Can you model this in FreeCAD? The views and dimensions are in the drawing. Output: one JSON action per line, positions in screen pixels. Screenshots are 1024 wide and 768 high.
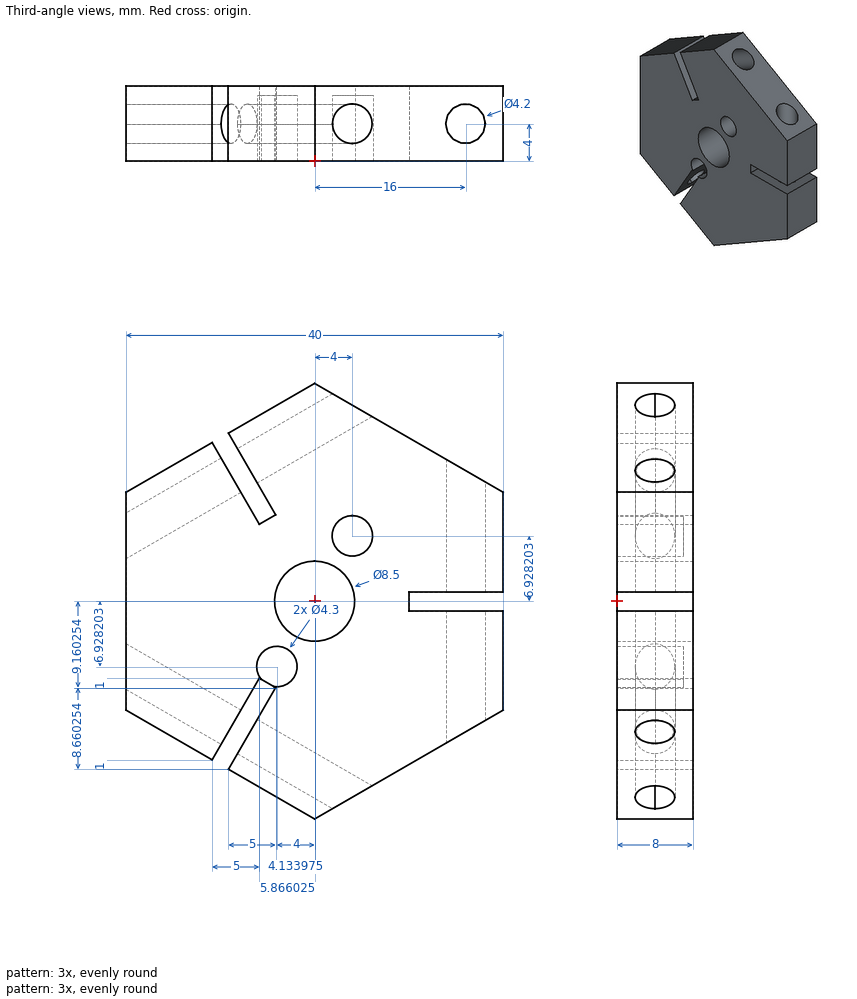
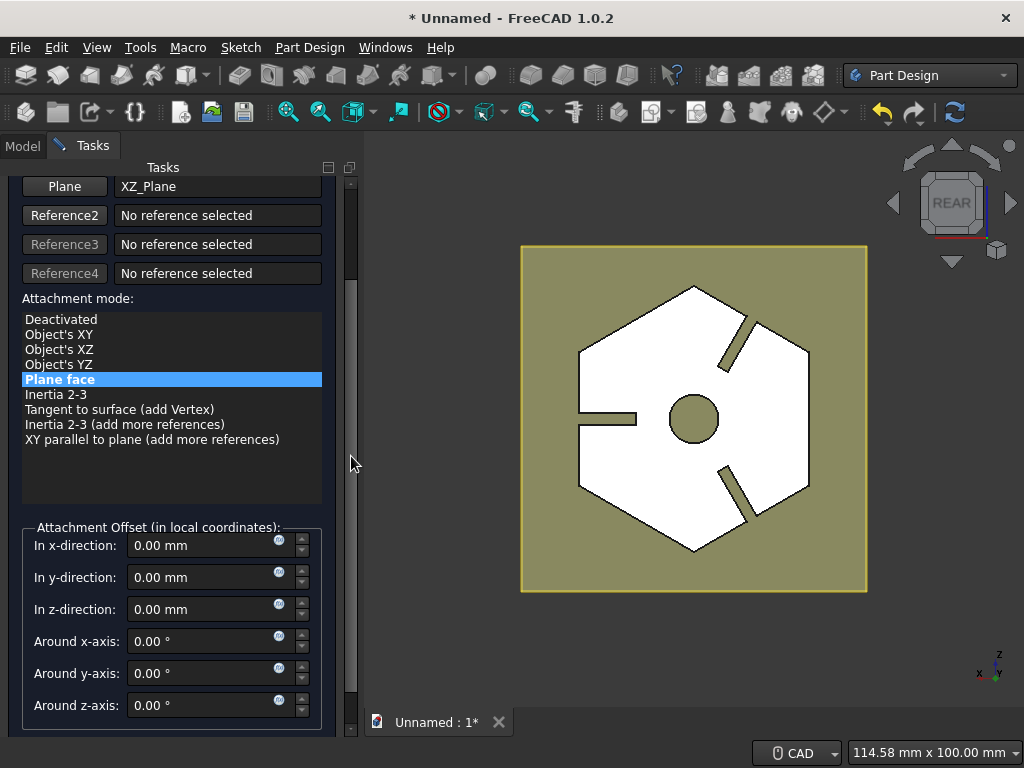
{"action": "triple_click", "coordinate": [210, 609]}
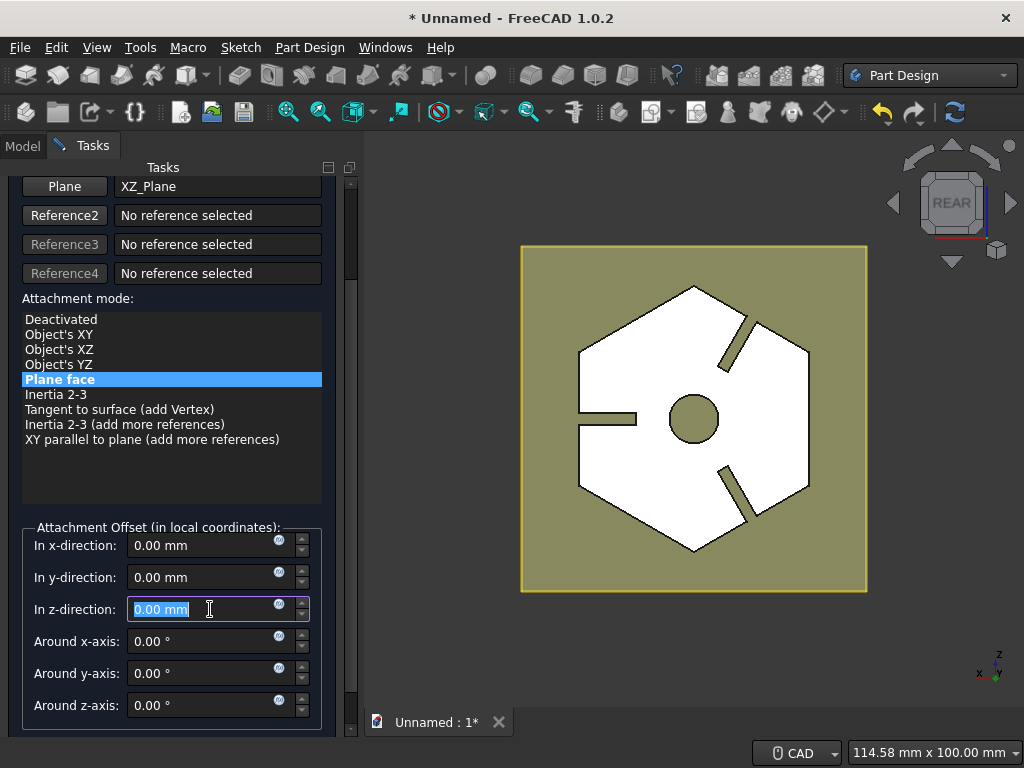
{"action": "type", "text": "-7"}
{"action": "key", "text": "Tab"}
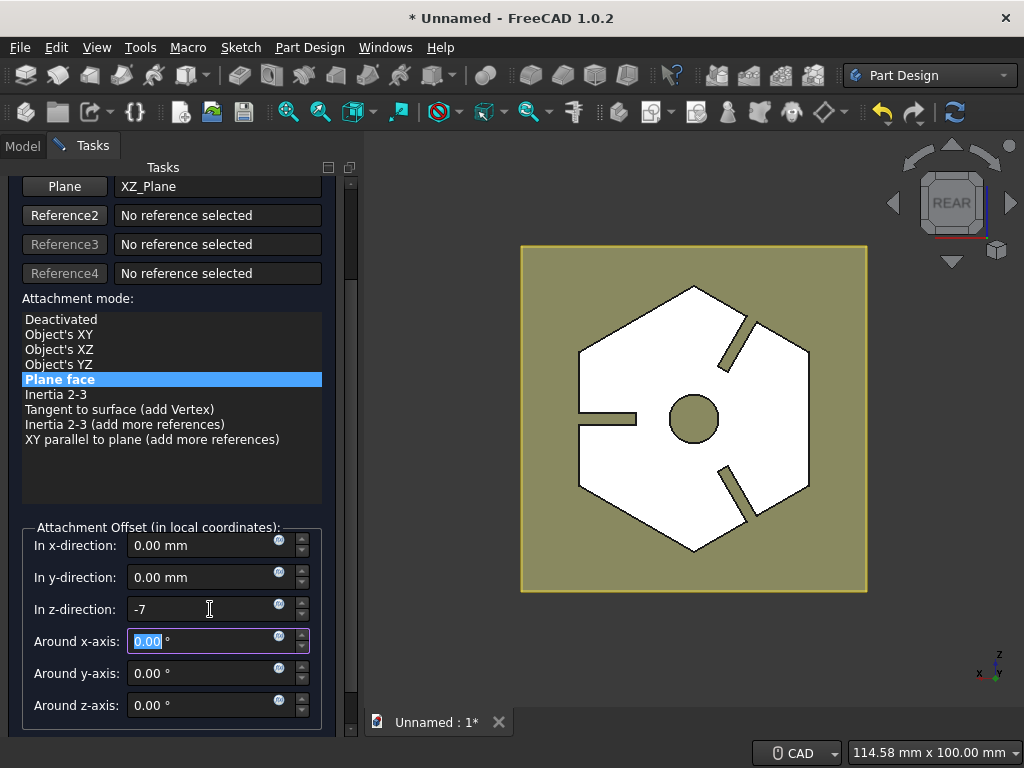
{"action": "scroll", "coordinate": [351, 456], "scroll_direction": "up", "scroll_amount": 3}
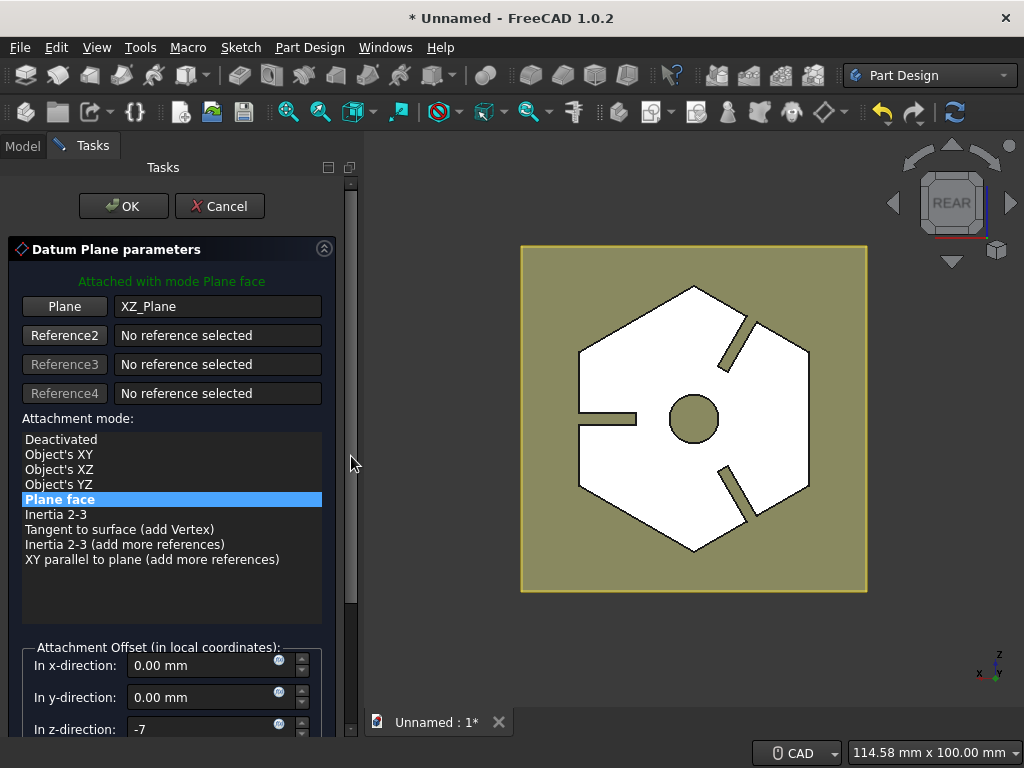
{"action": "left_click", "coordinate": [124, 206]}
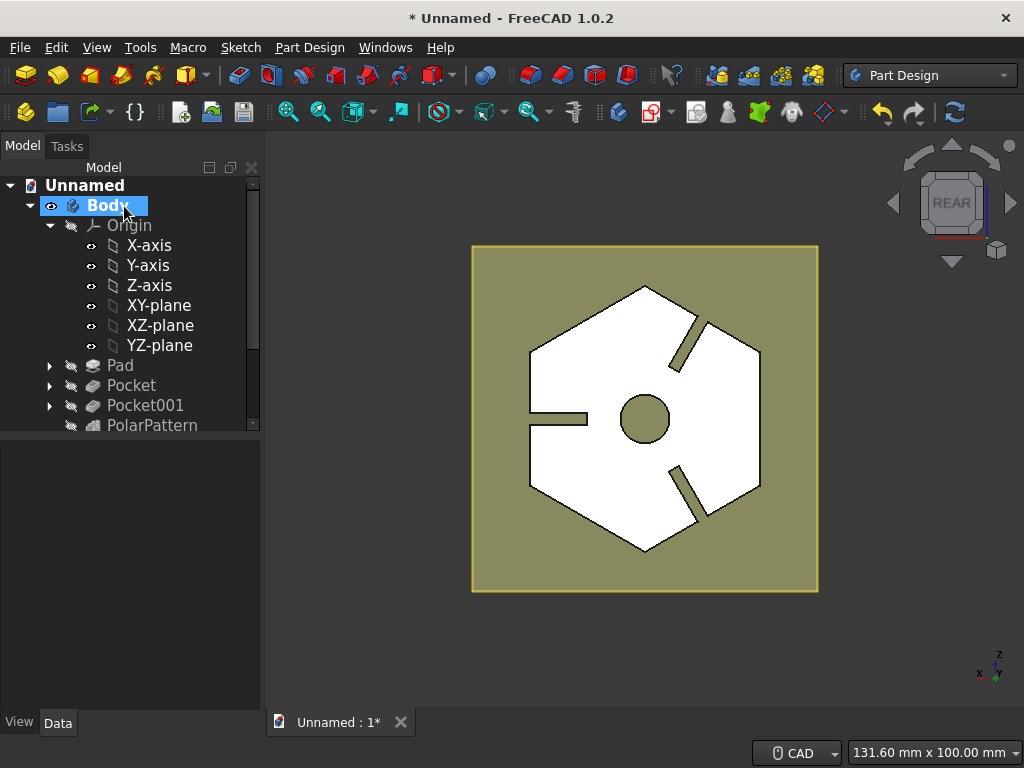
{"action": "scroll", "coordinate": [100, 301], "scroll_direction": "down", "scroll_amount": 3}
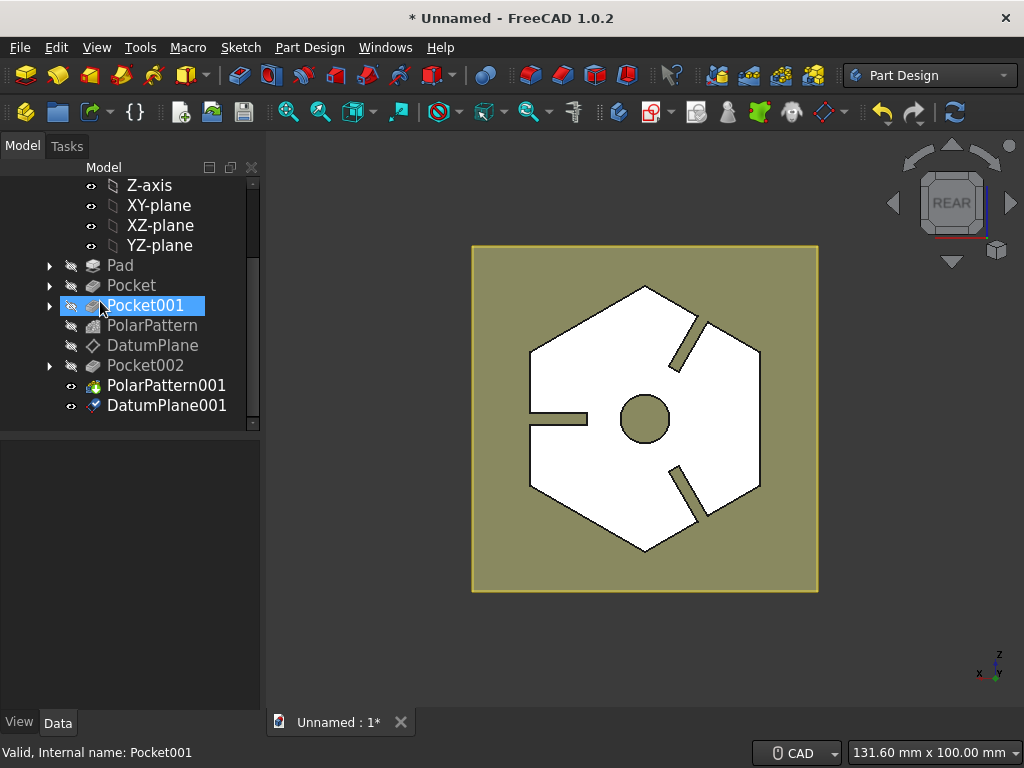
{"action": "left_click", "coordinate": [116, 406]}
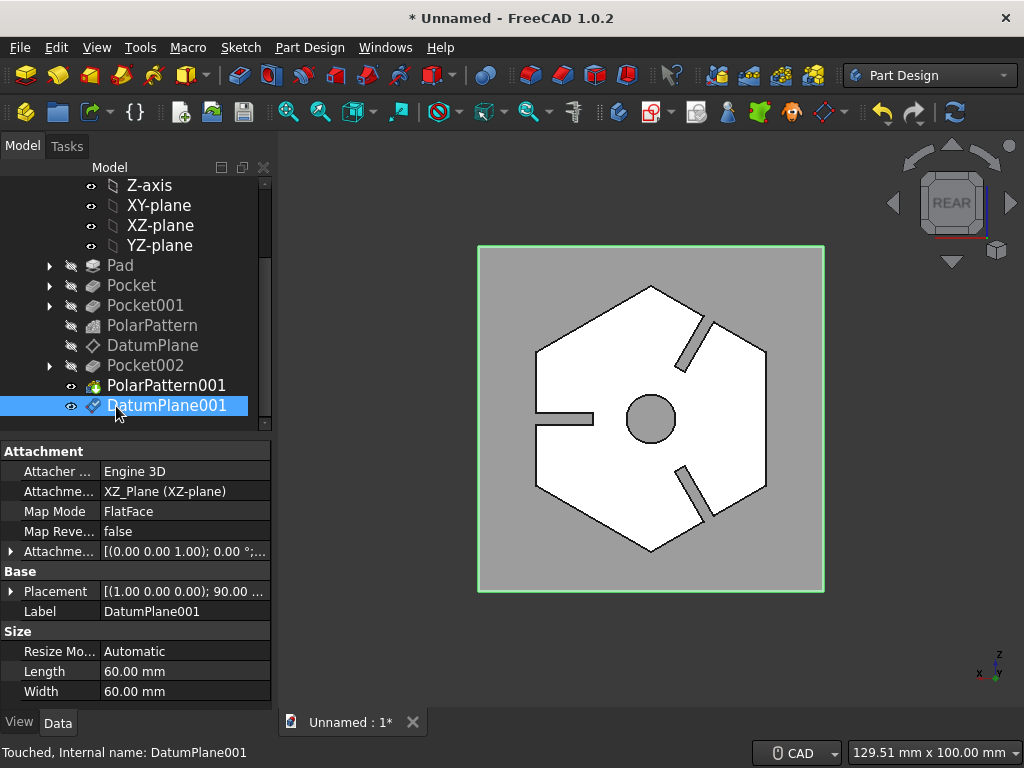
{"action": "left_click", "coordinate": [652, 112]}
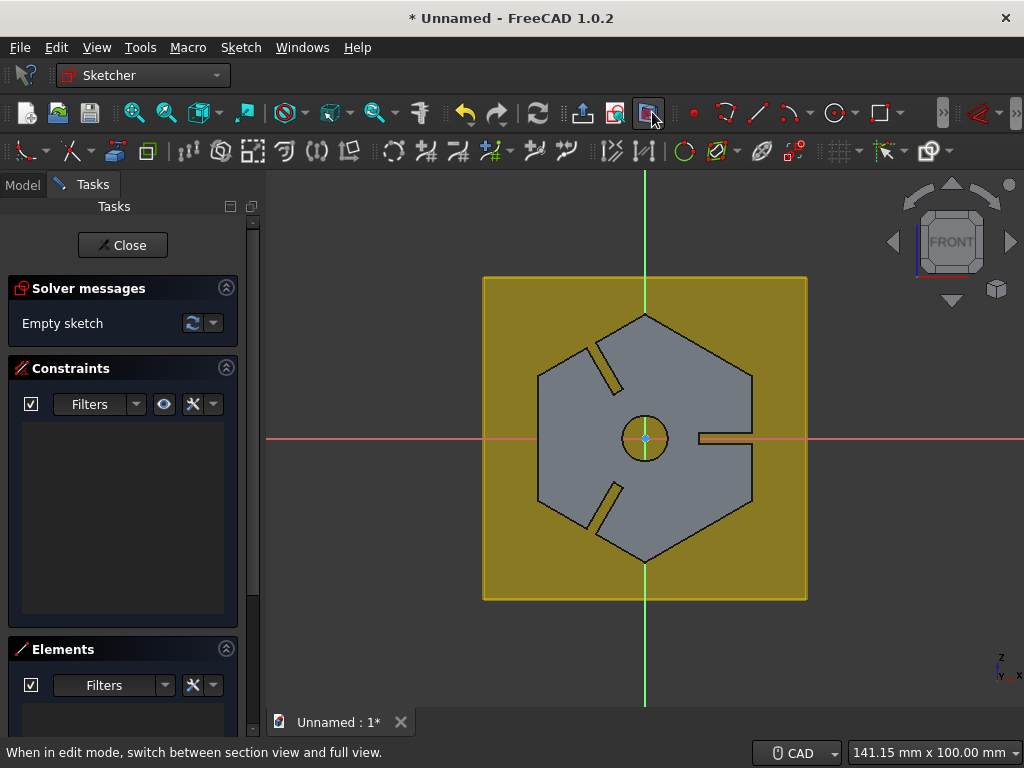
{"action": "key", "text": "q s"}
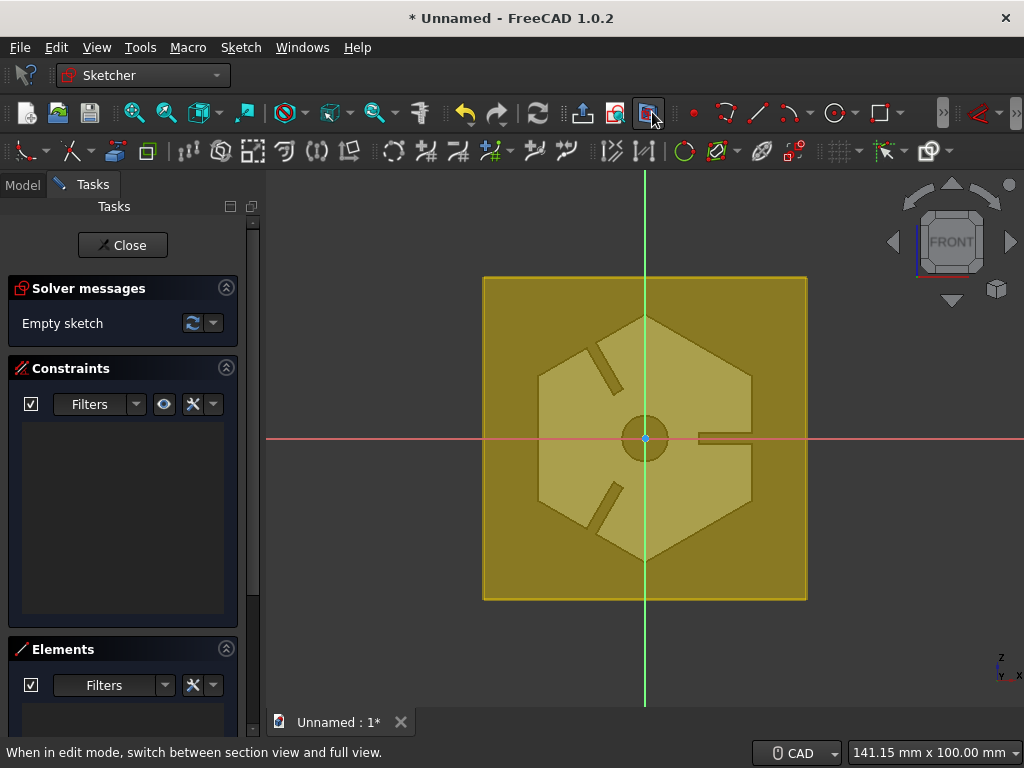
{"action": "scroll", "coordinate": [675, 439], "scroll_direction": "up", "scroll_amount": 6}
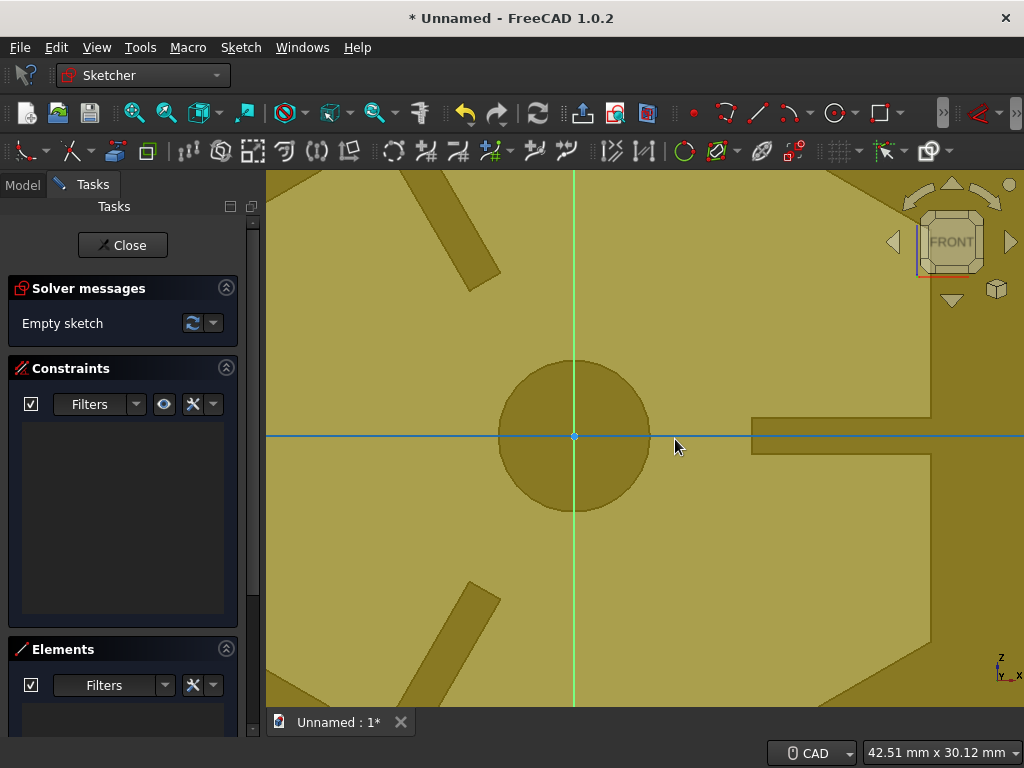
{"action": "key", "text": "g c"}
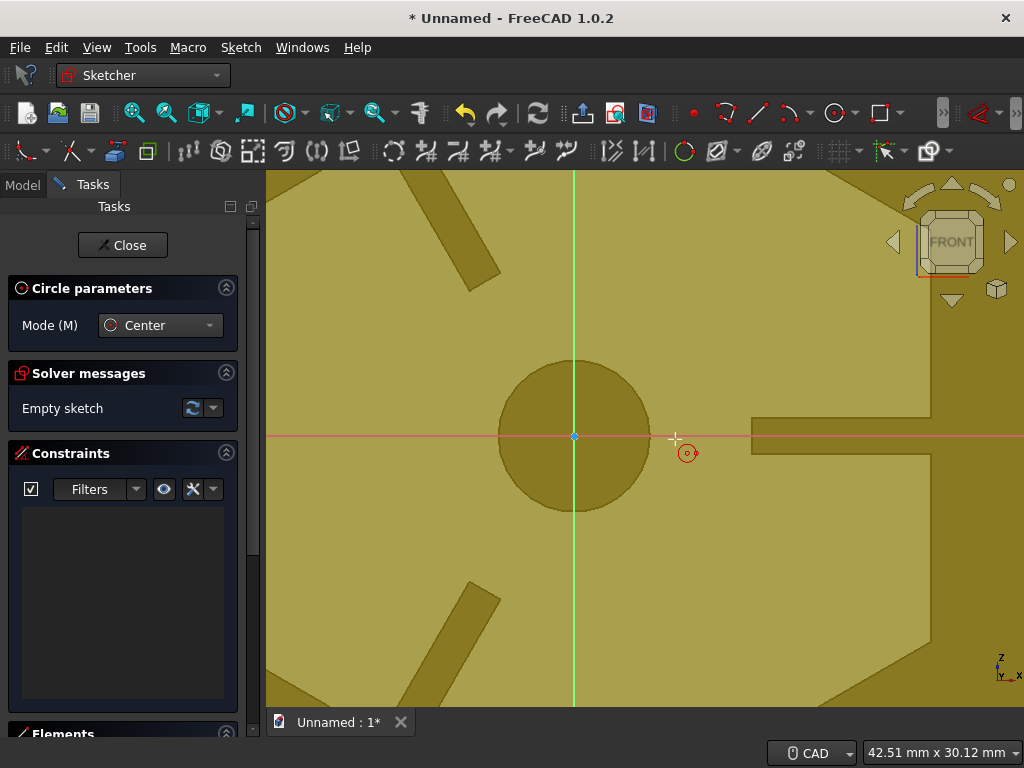
{"action": "left_click", "coordinate": [503, 560]}
{"action": "mouse_move", "coordinate": [530, 533]}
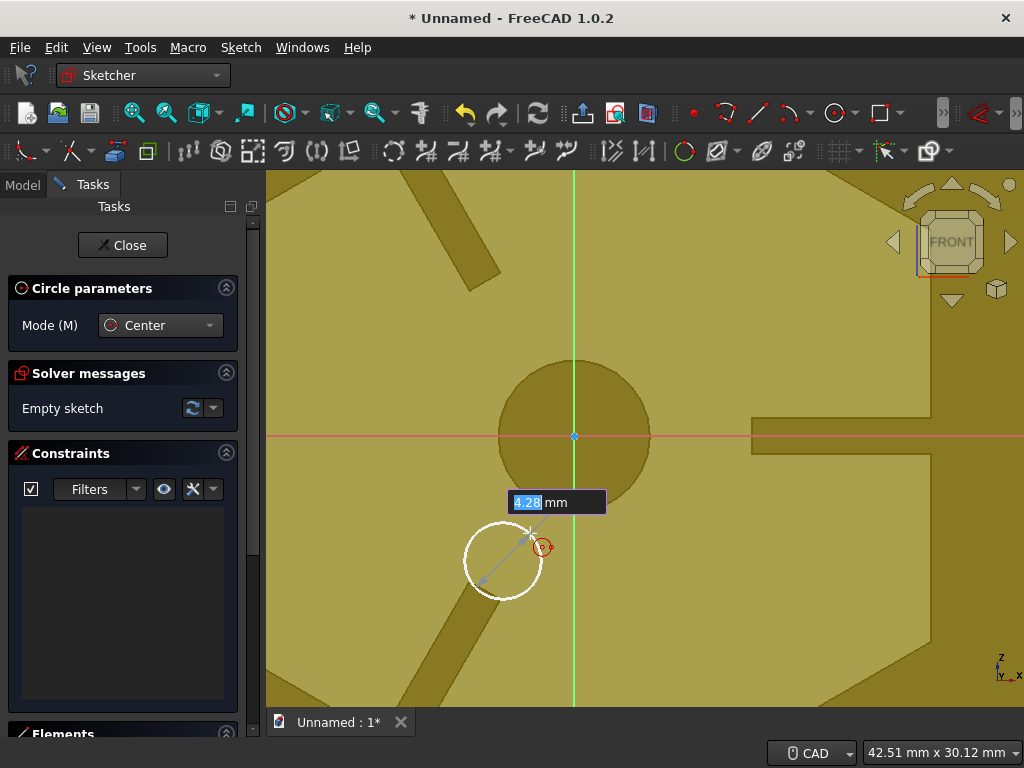
{"action": "type", "text": "4.3"}
{"action": "key", "text": "Return"}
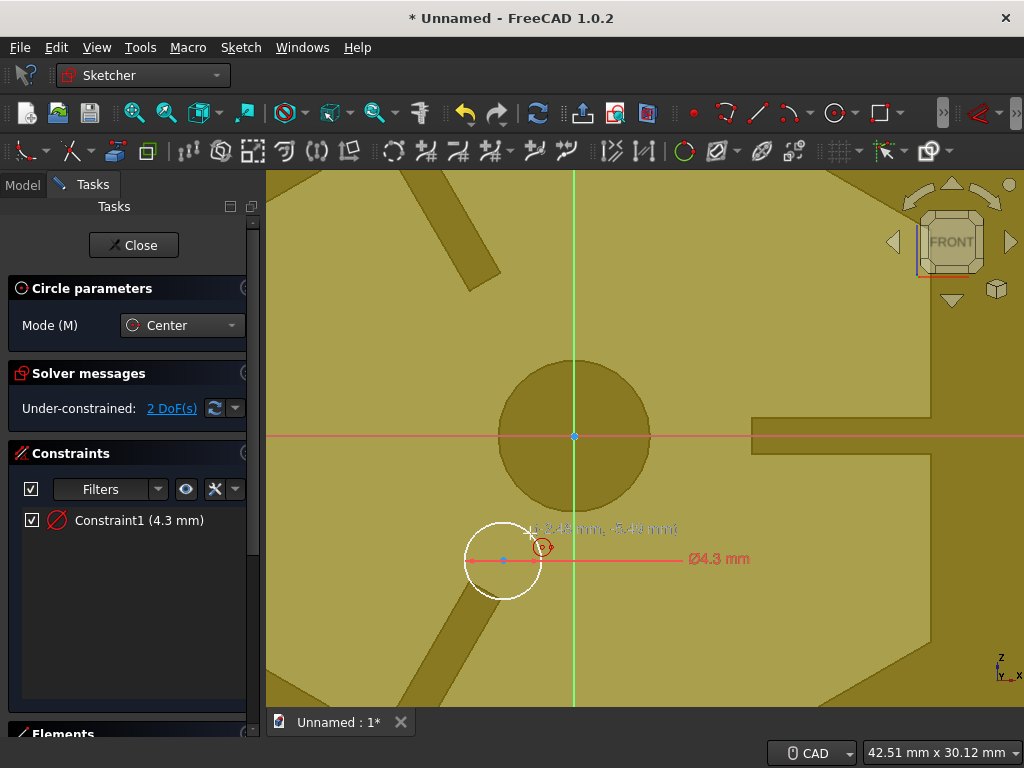
{"action": "left_click", "coordinate": [645, 313]}
{"action": "mouse_move", "coordinate": [673, 286]}